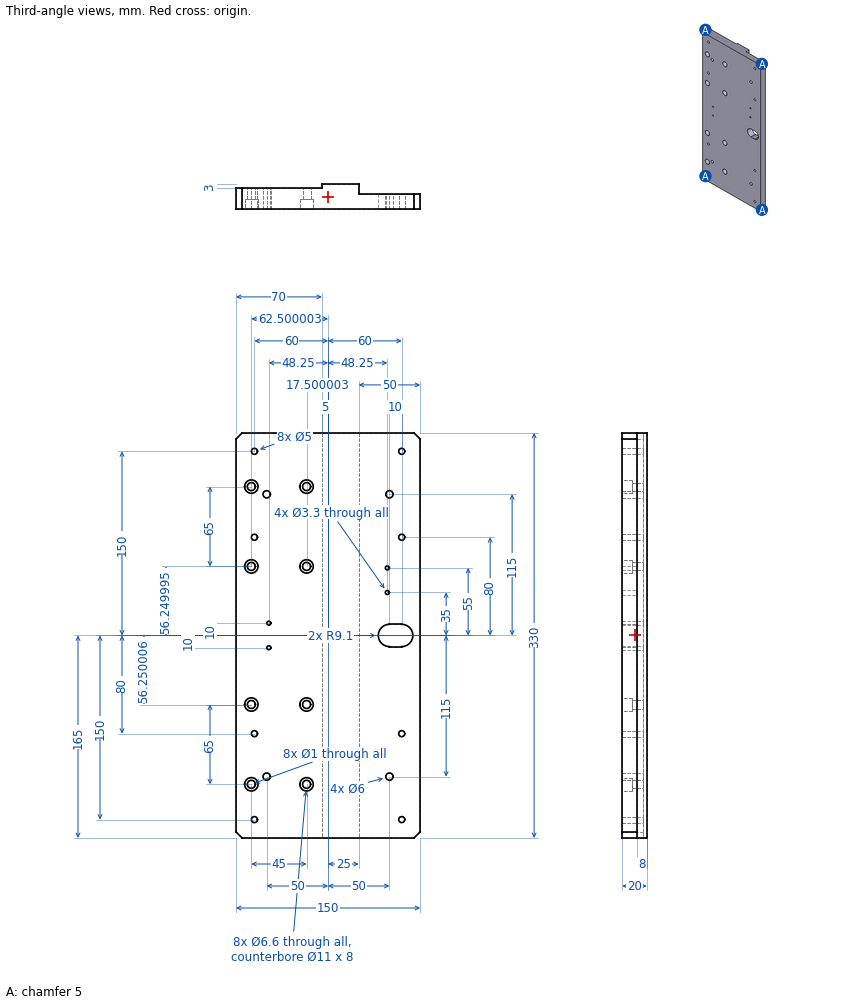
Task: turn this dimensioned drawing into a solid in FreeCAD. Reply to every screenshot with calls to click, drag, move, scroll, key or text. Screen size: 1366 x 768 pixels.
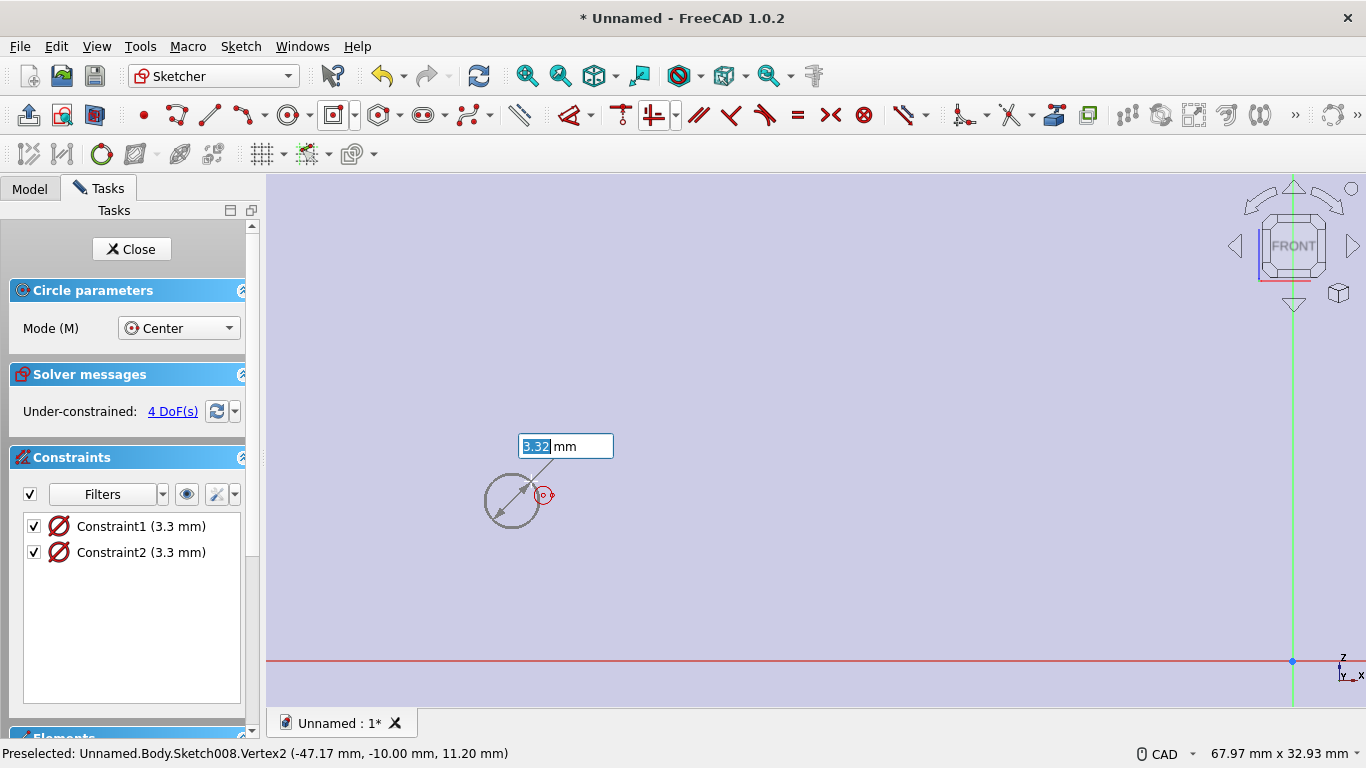
text(3.3)
key(Return)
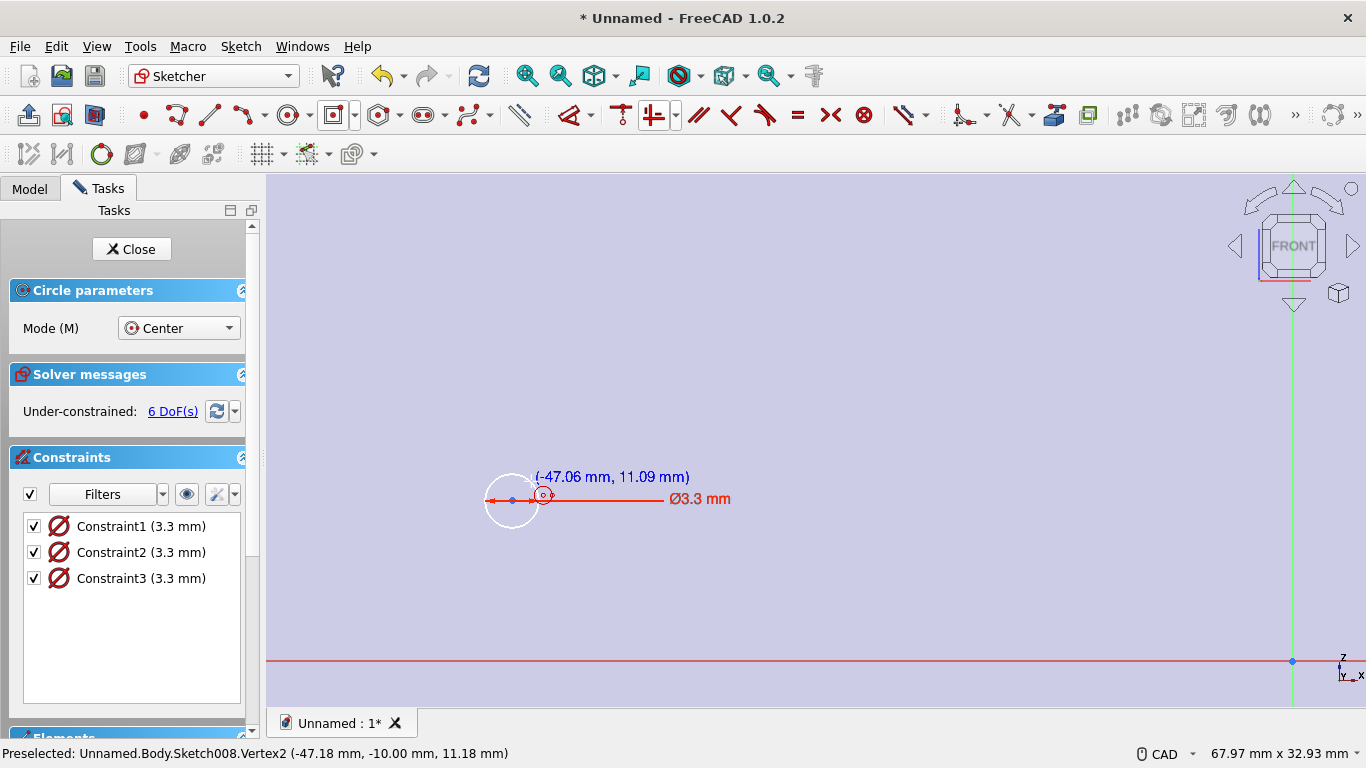
scroll(513, 502, down, 6)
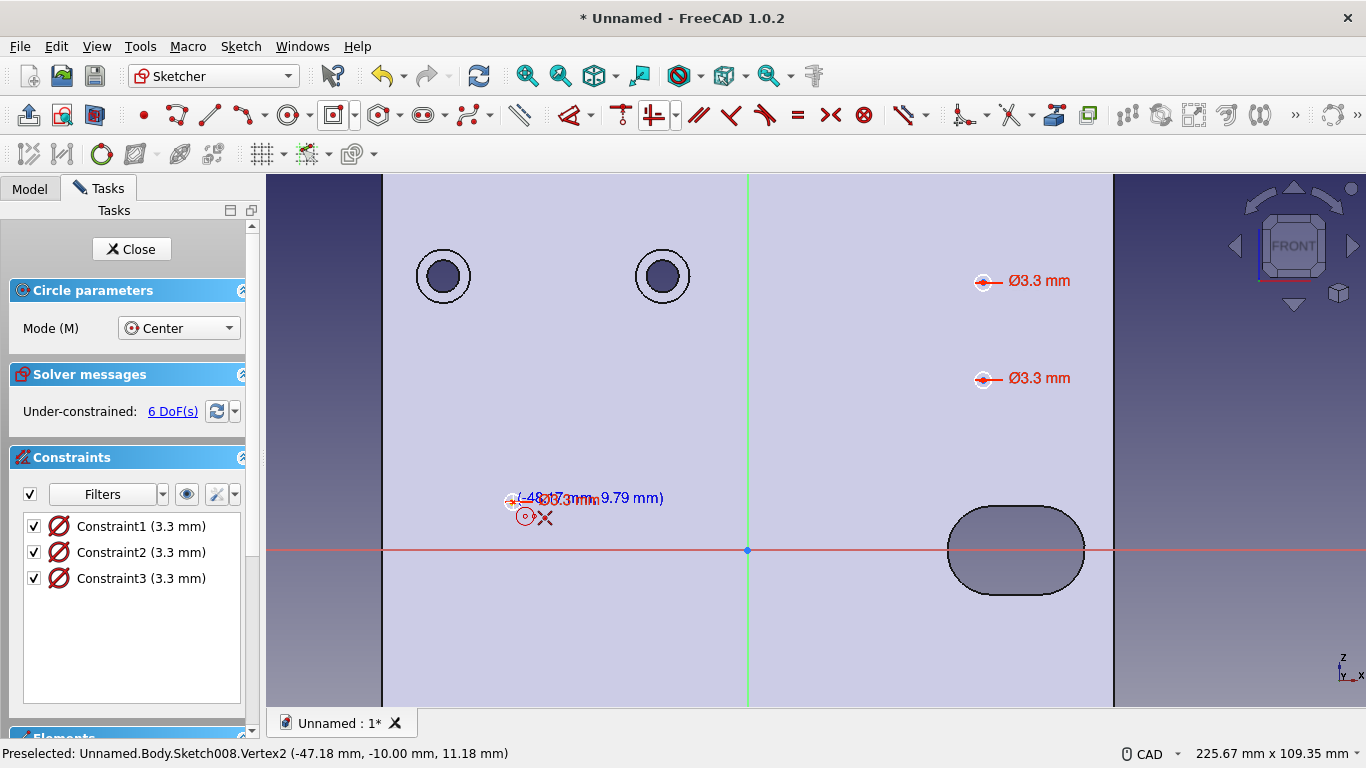
scroll(513, 599, up, 6)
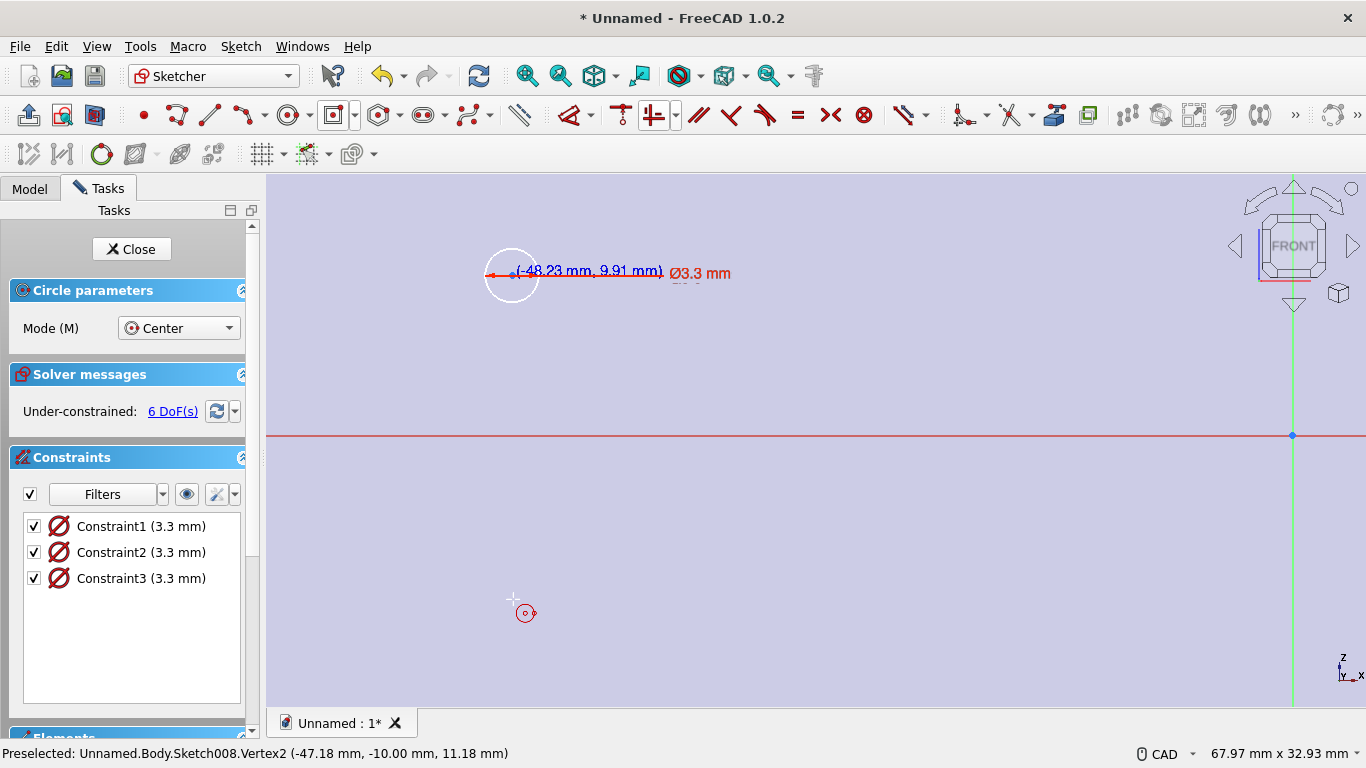
click(512, 598)
move(531, 579)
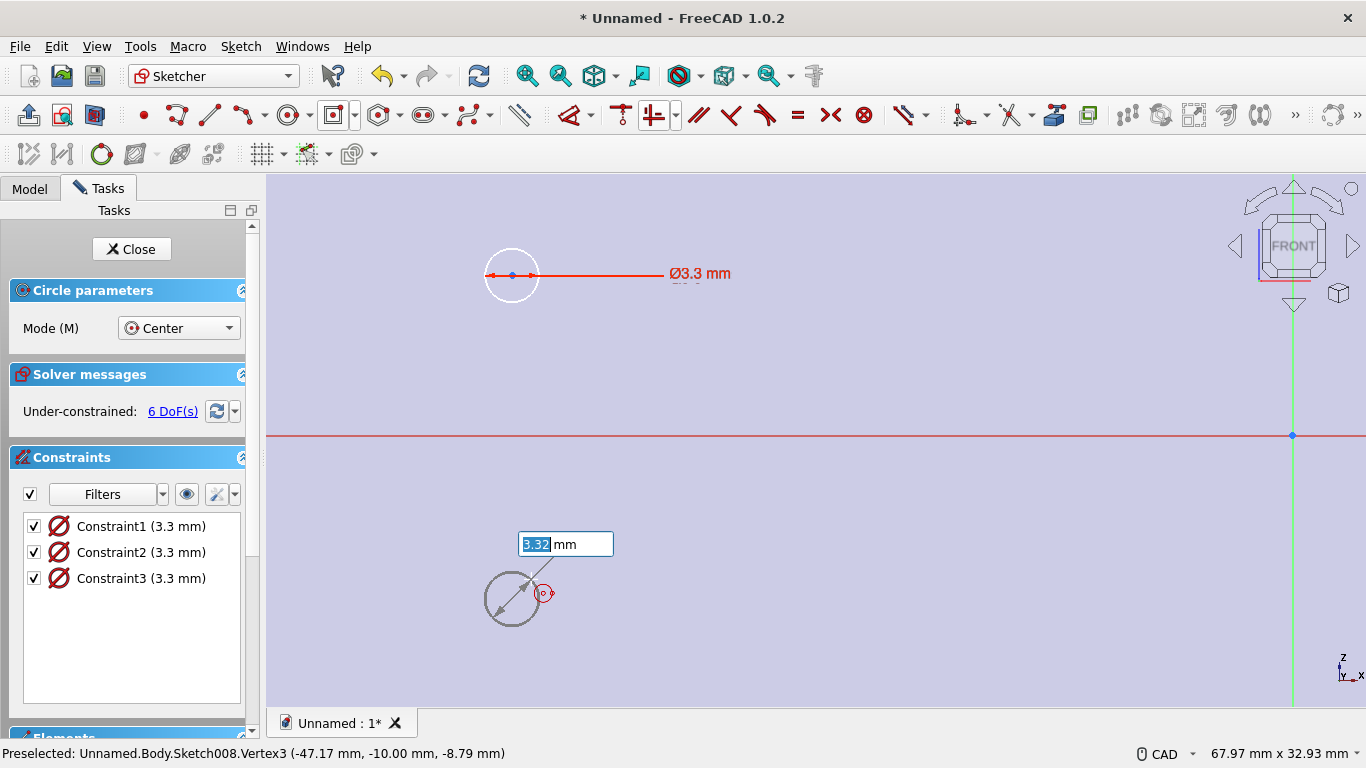
text(3.3)
key(Return)
key(Escape)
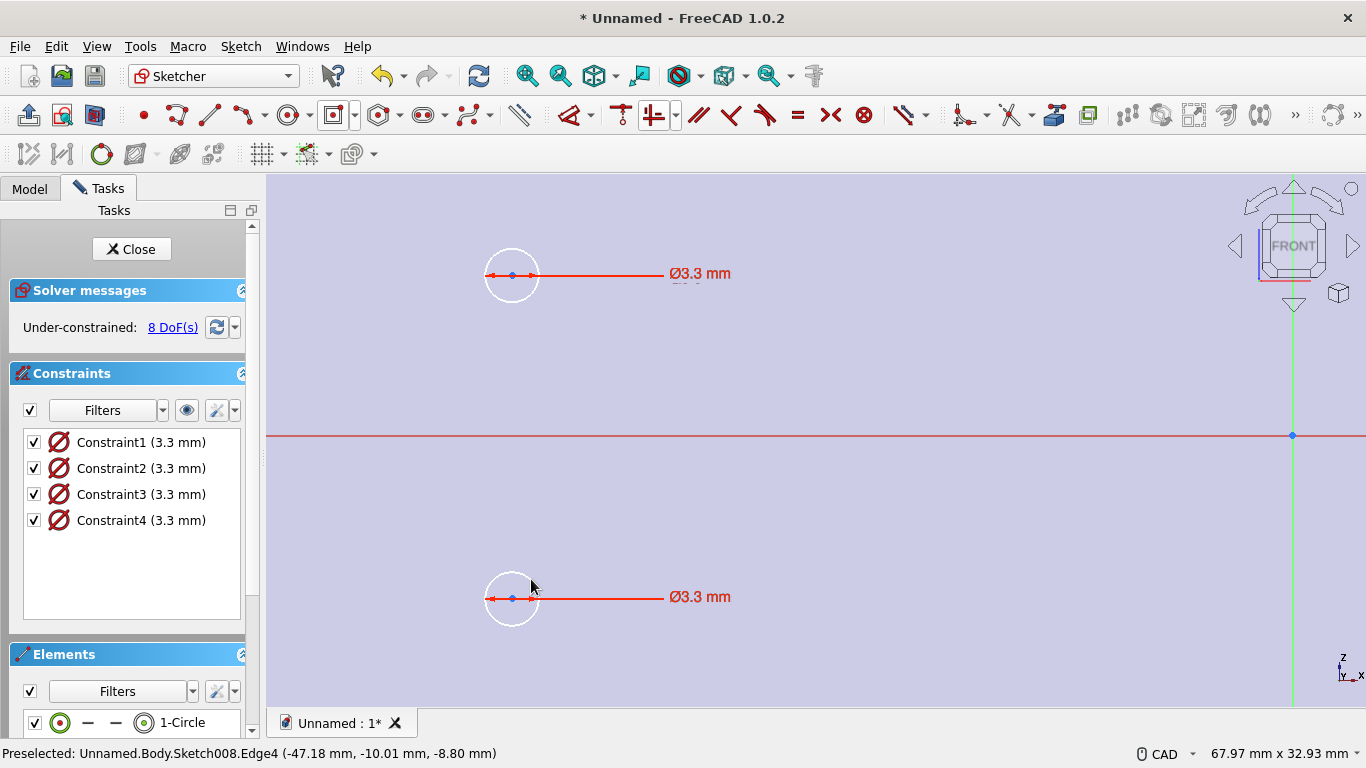
scroll(513, 599, down, 6)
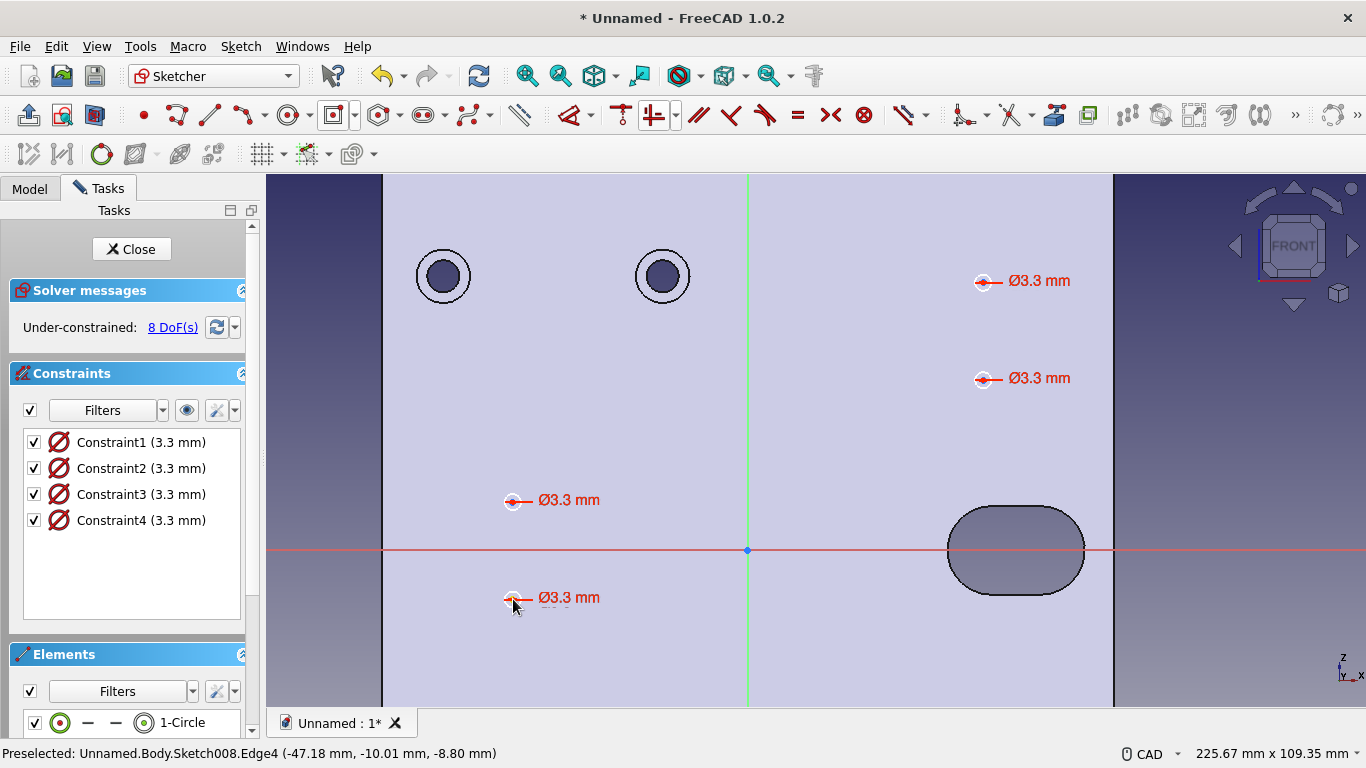
click(983, 380)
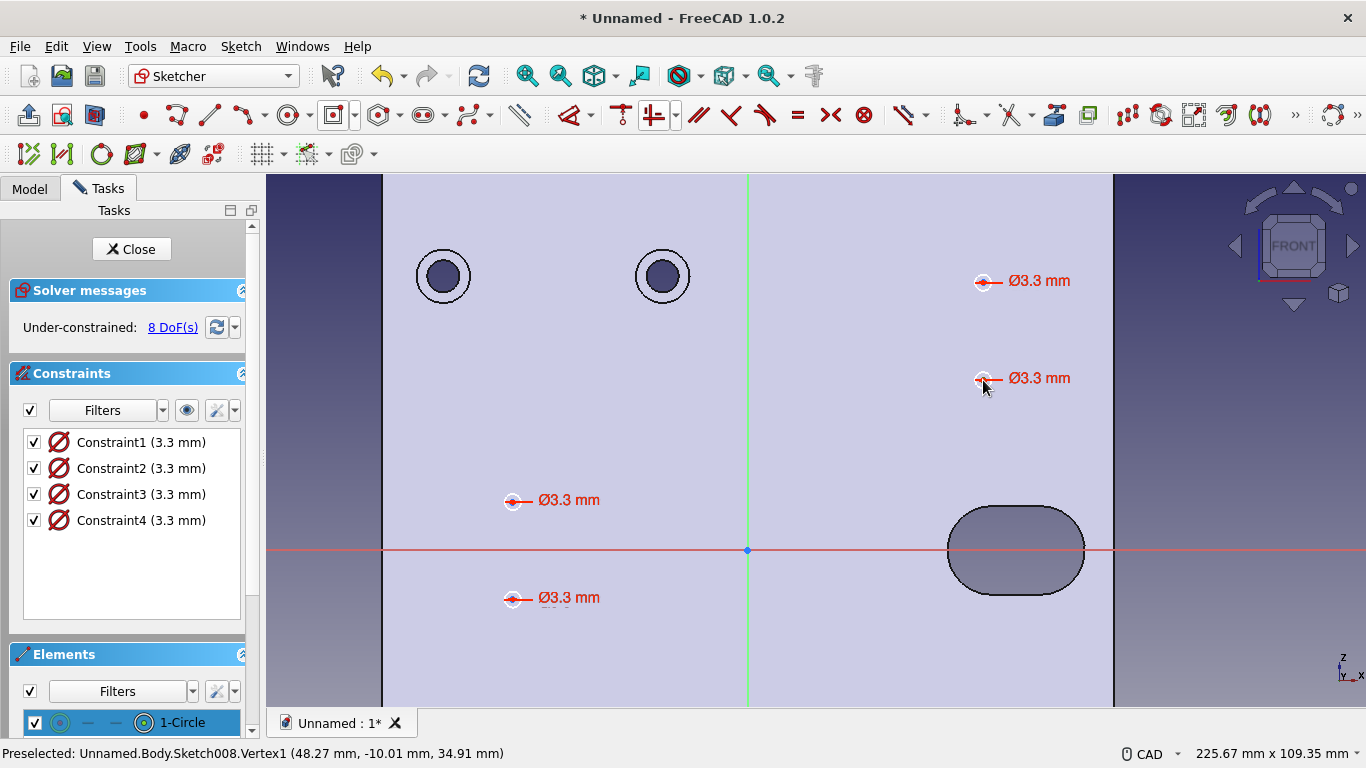
click(983, 283)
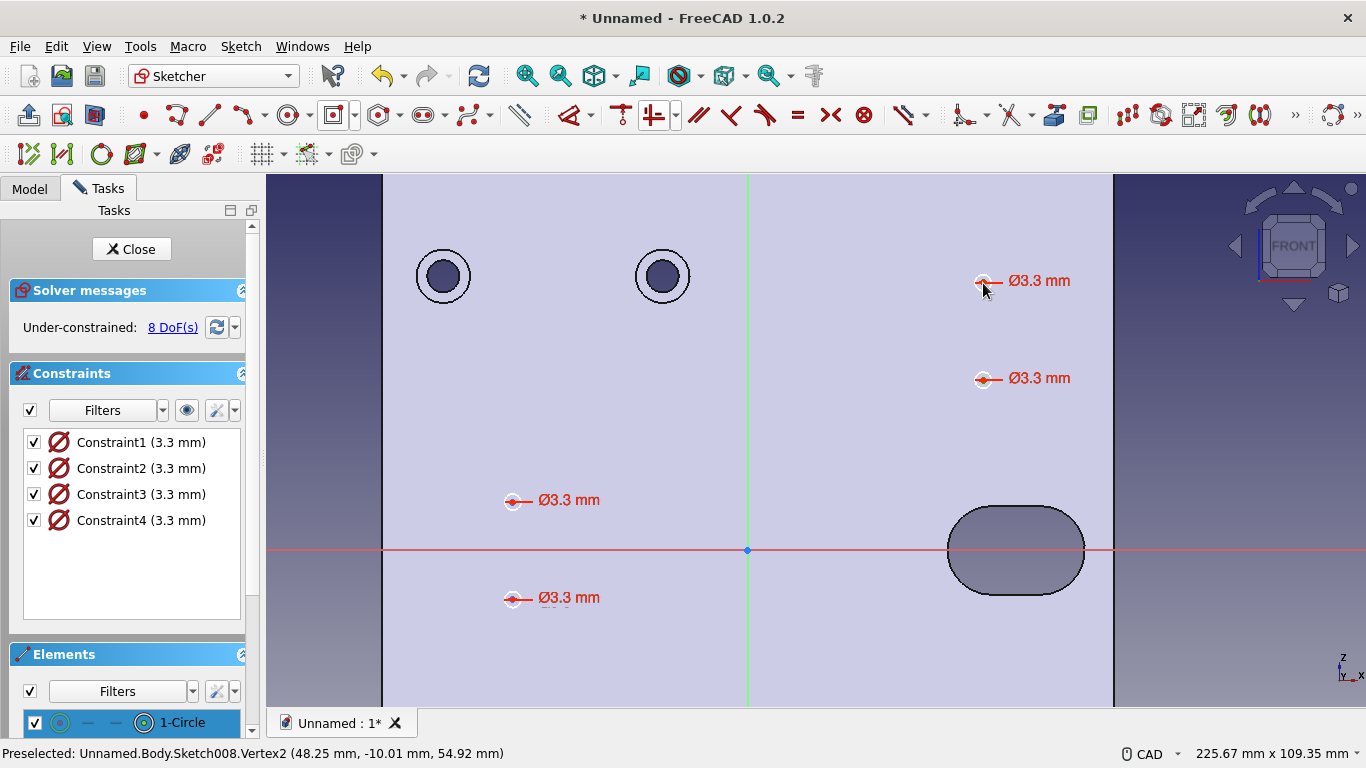
click(676, 116)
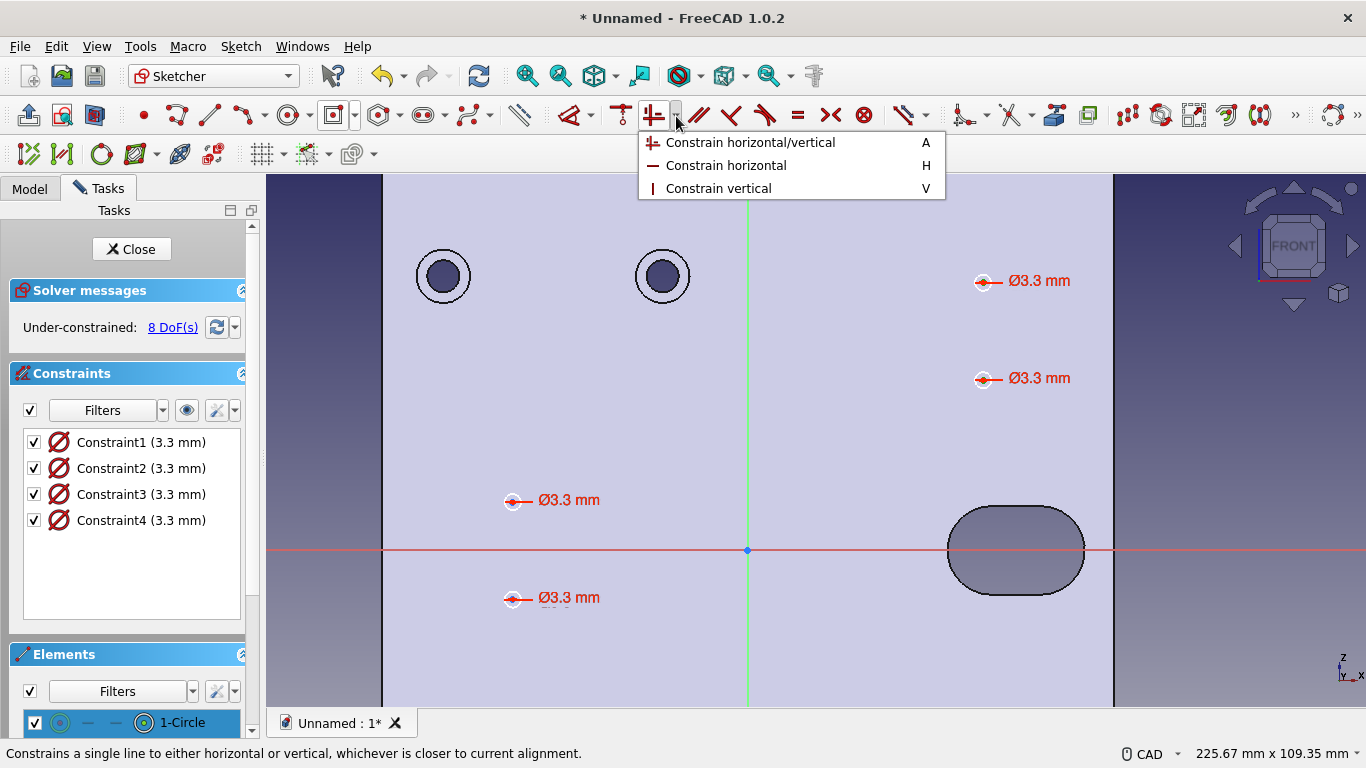
click(792, 188)